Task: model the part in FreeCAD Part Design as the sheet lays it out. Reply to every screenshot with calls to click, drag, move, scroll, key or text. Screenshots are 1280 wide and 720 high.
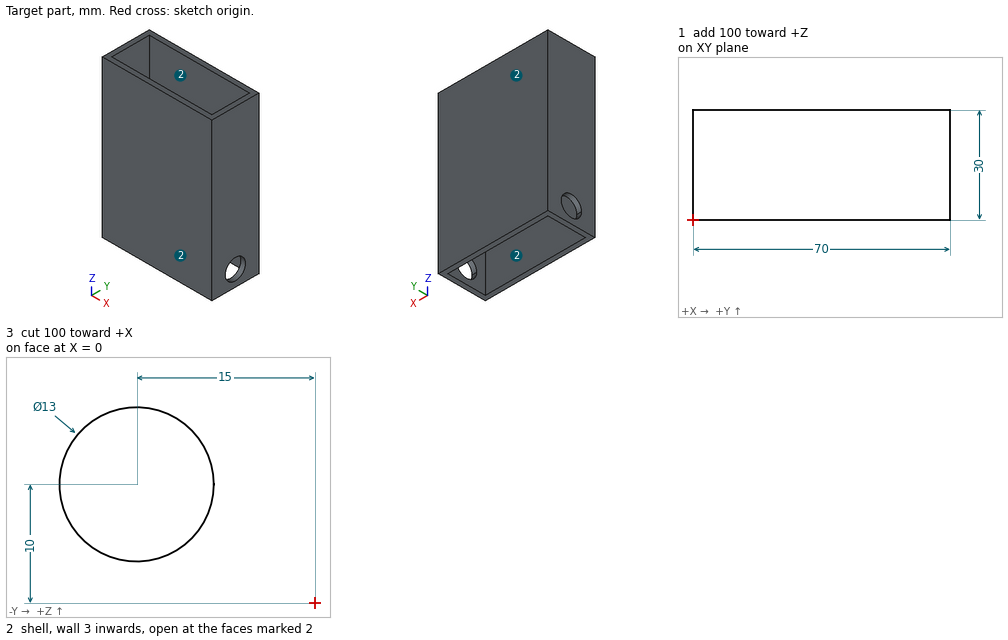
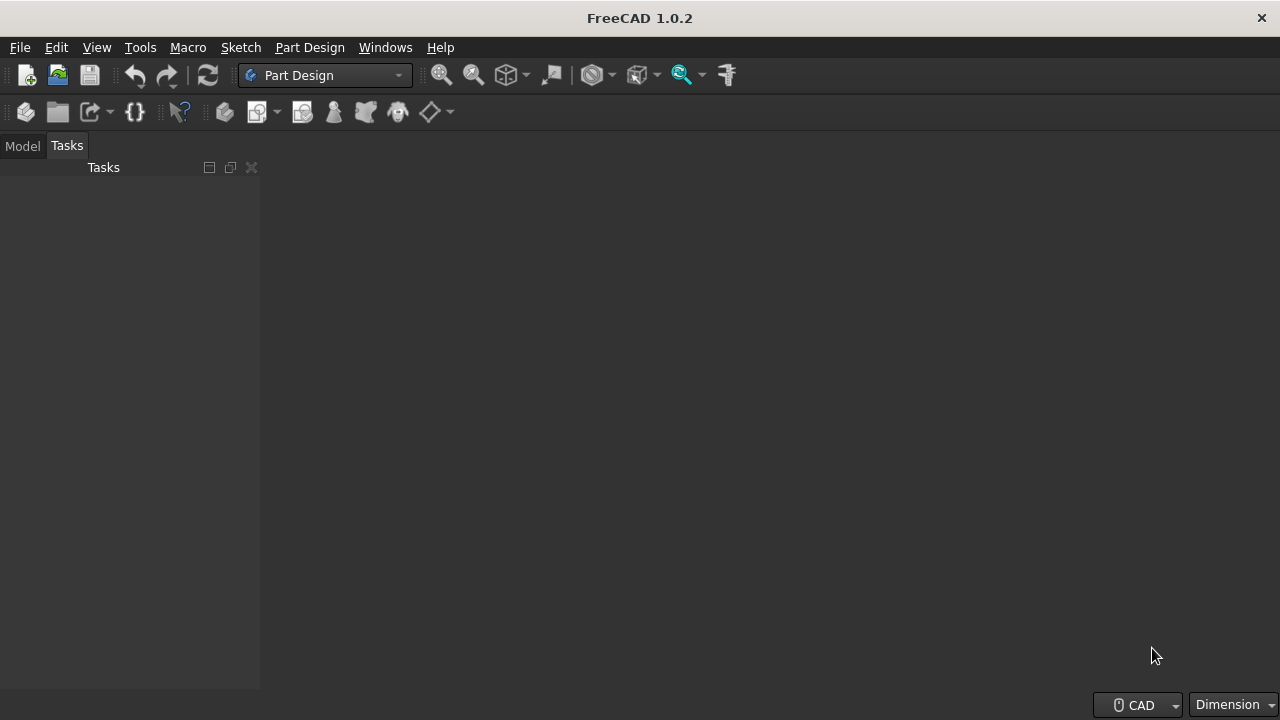
click(26, 76)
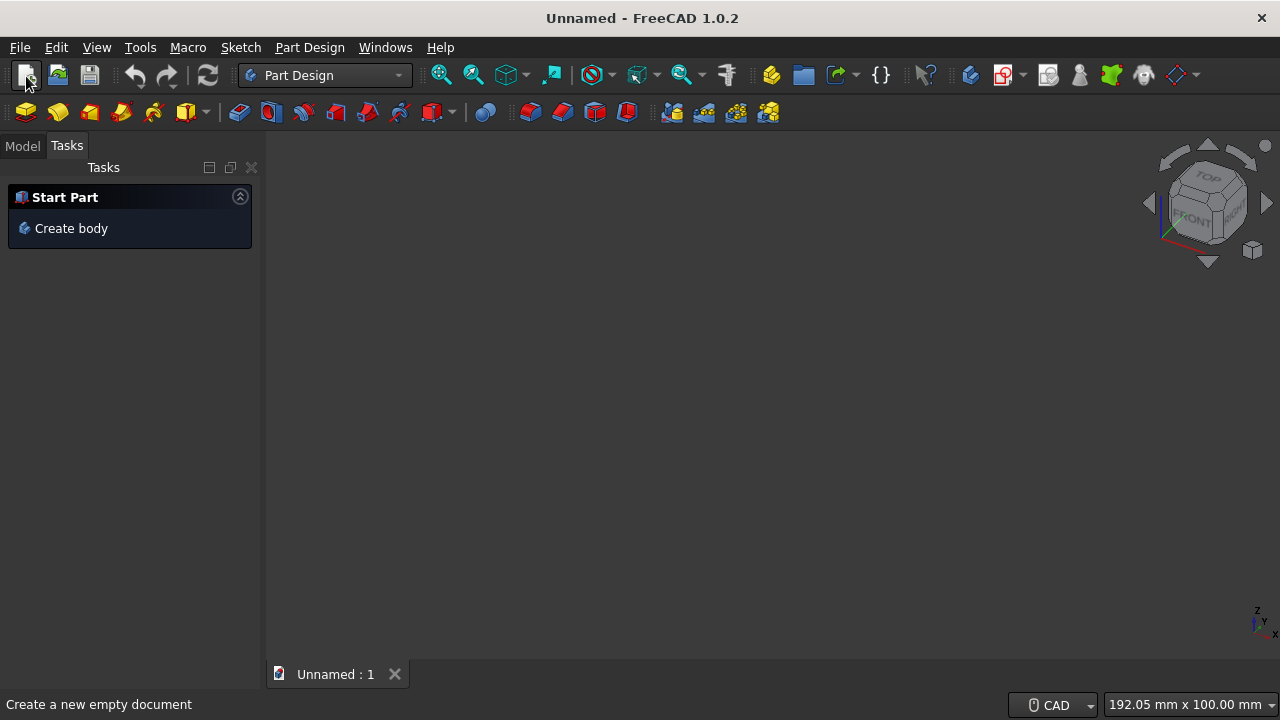
click(1004, 76)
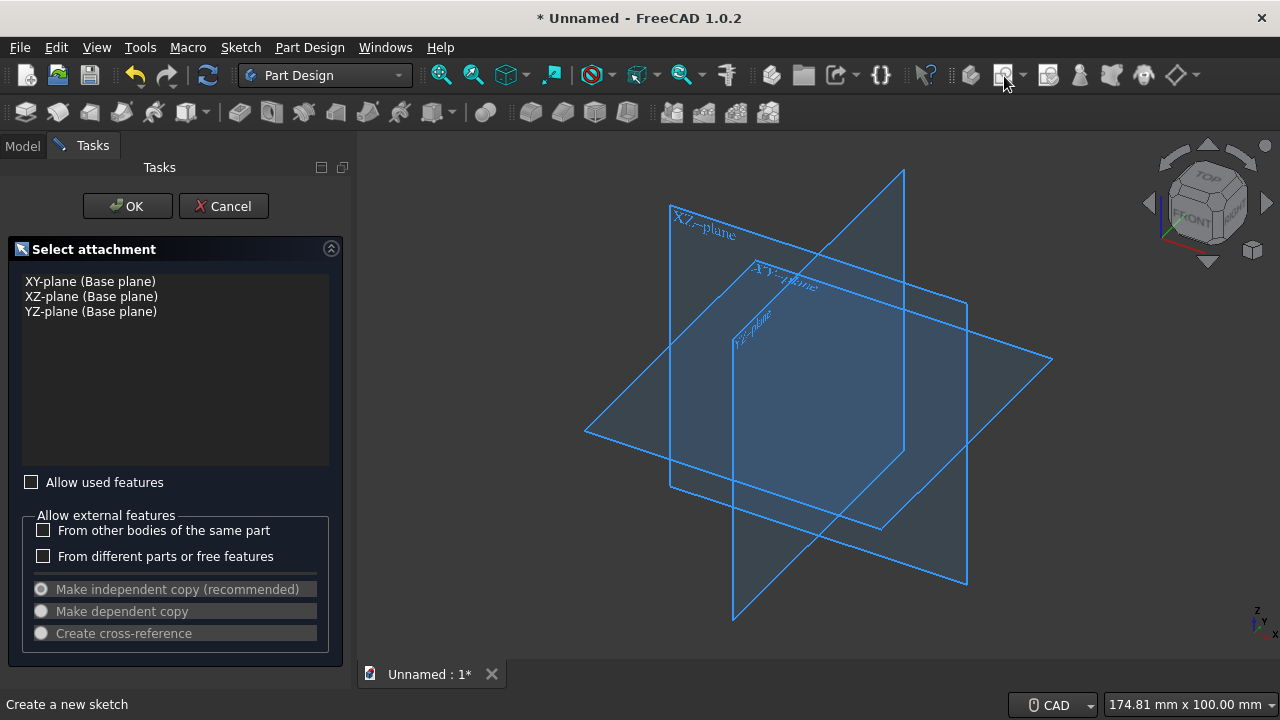
click(82, 282)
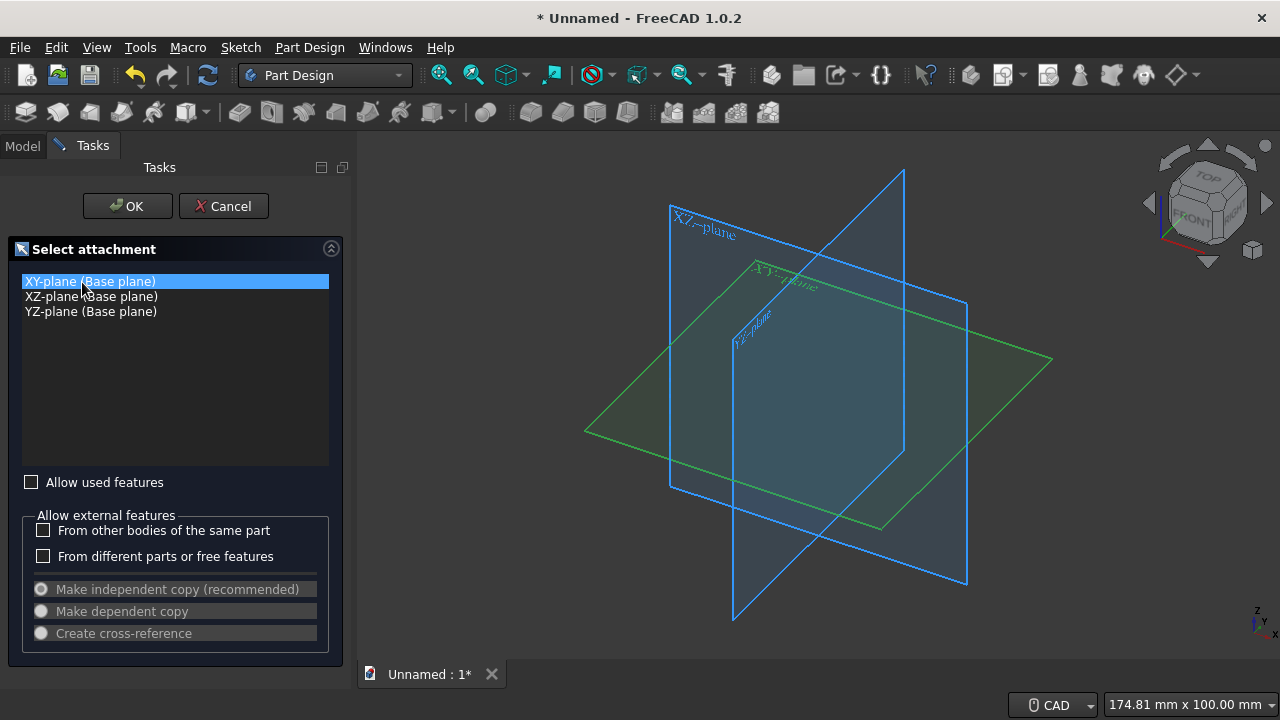
click(128, 206)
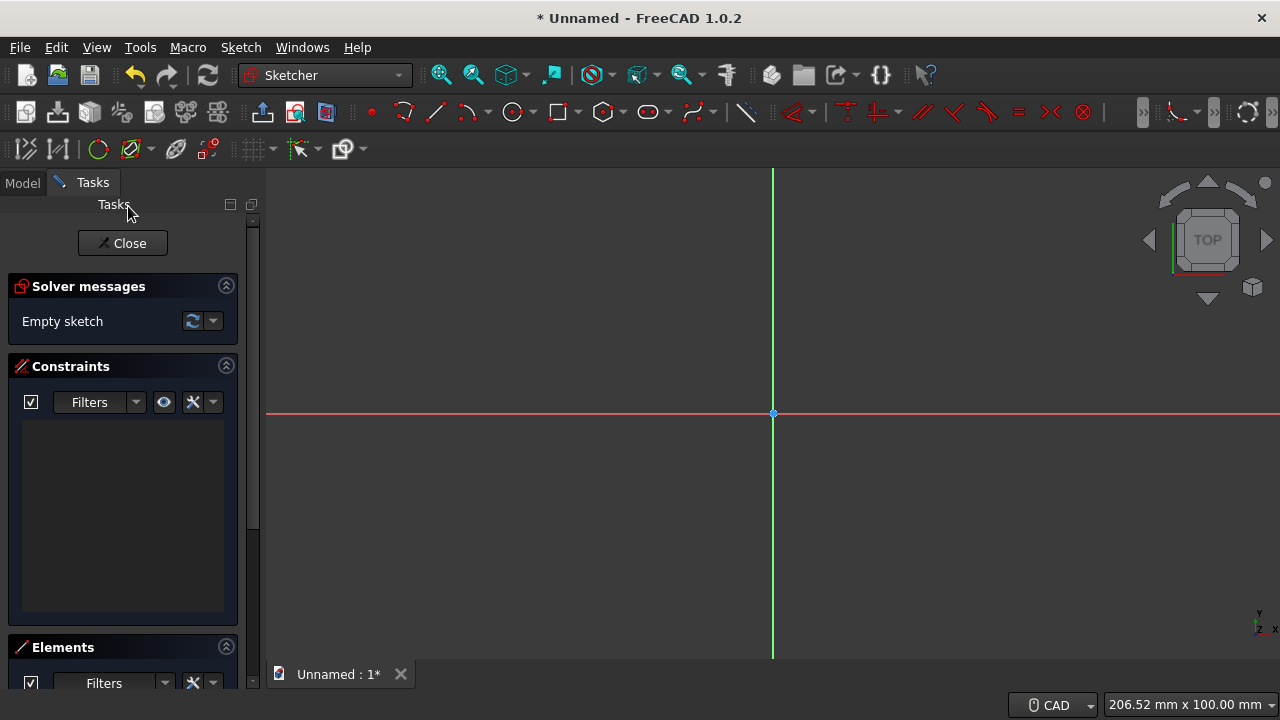
scroll(704, 414, down, 5)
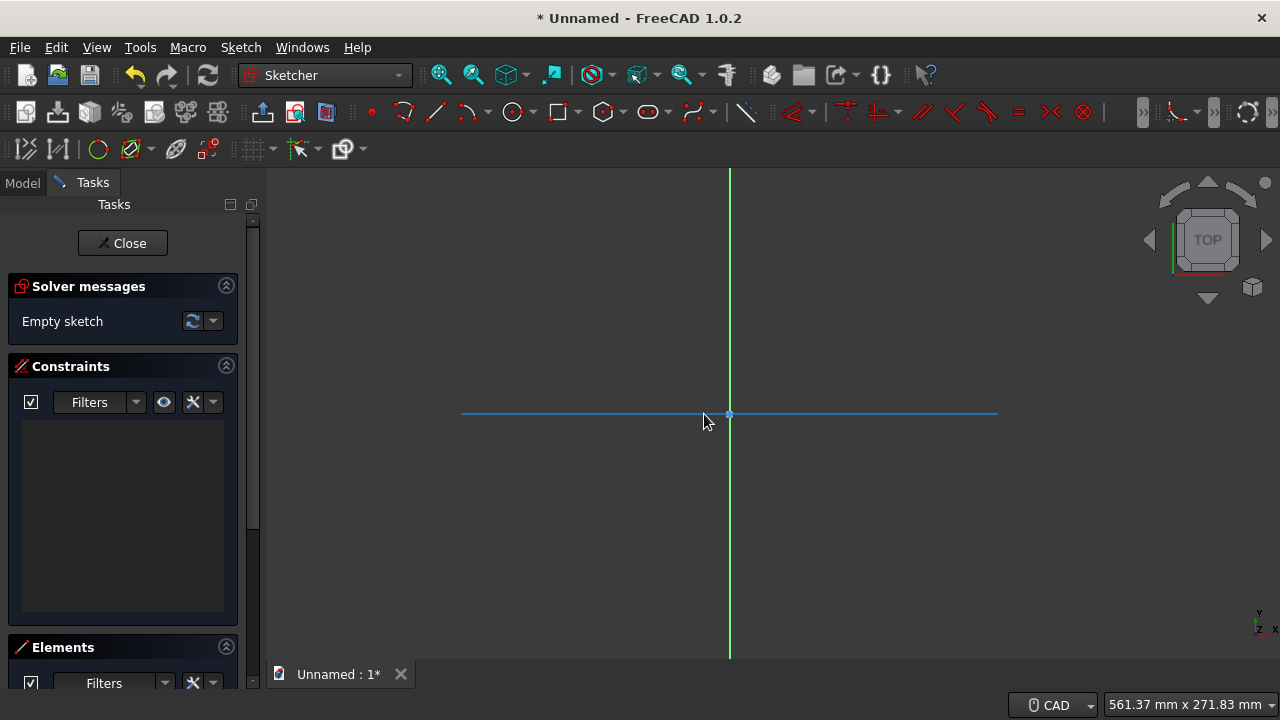
scroll(815, 380, up, 8)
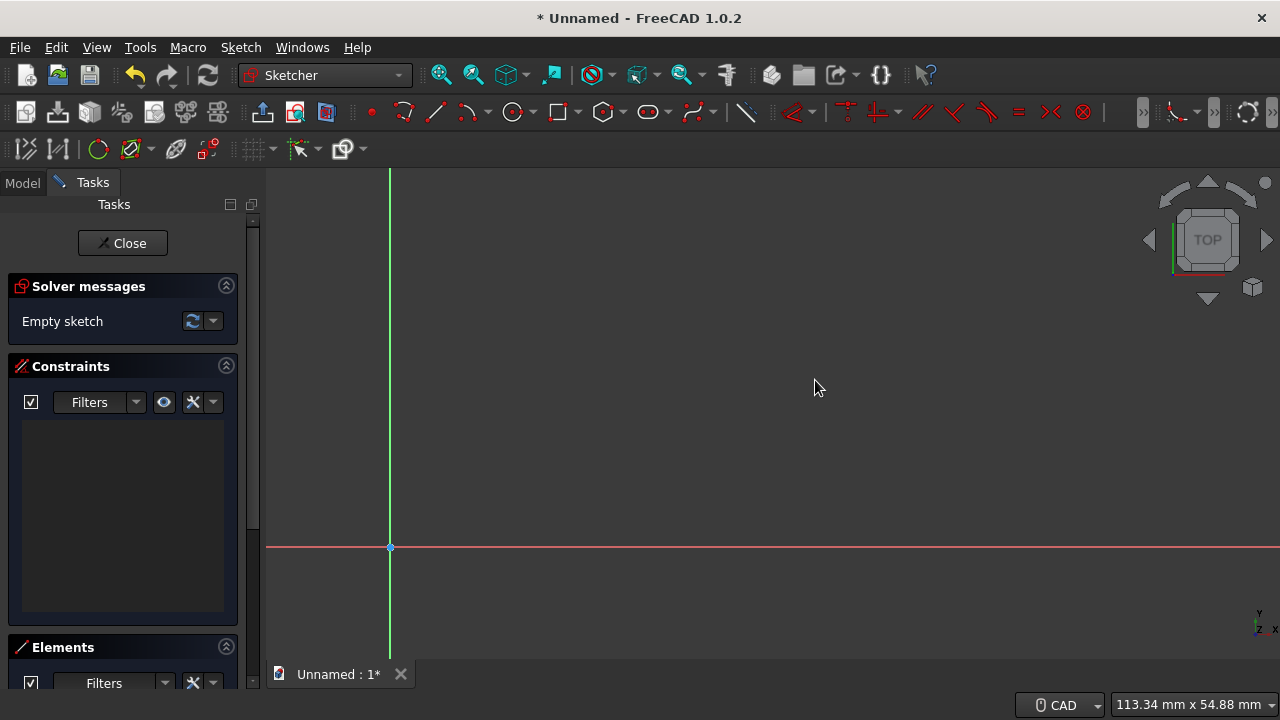
click(558, 112)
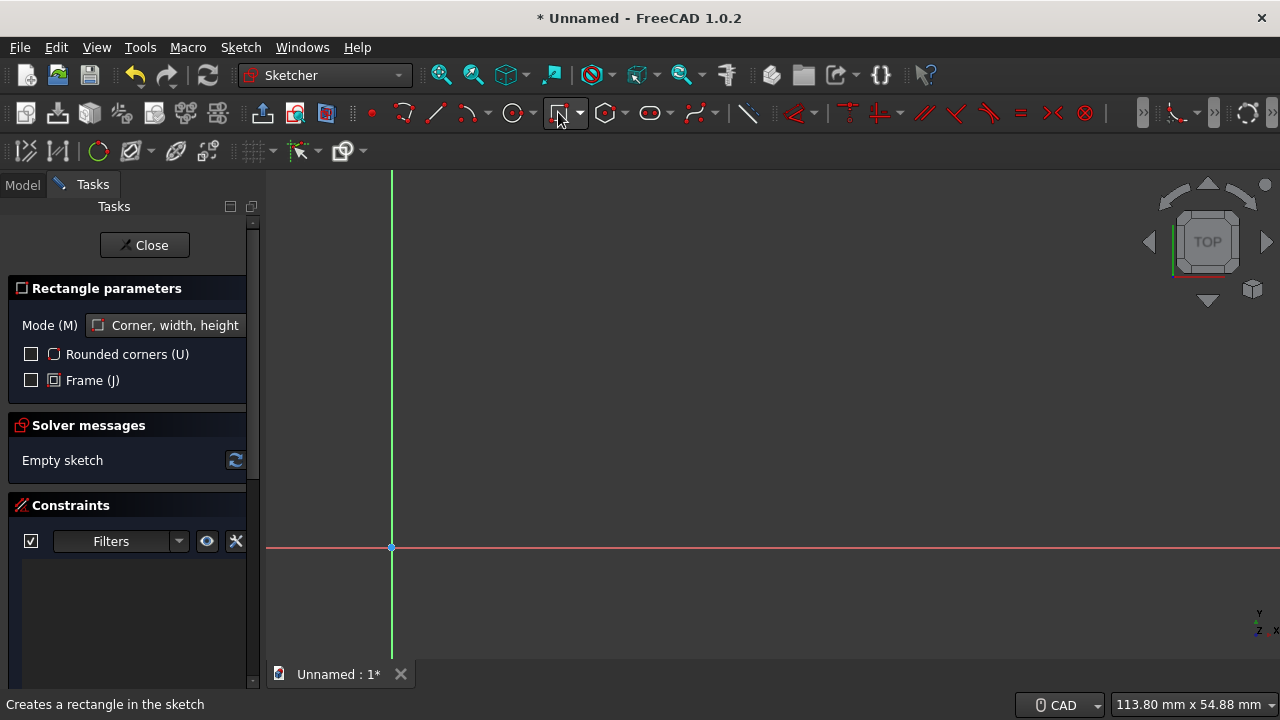
click(392, 548)
move(1015, 281)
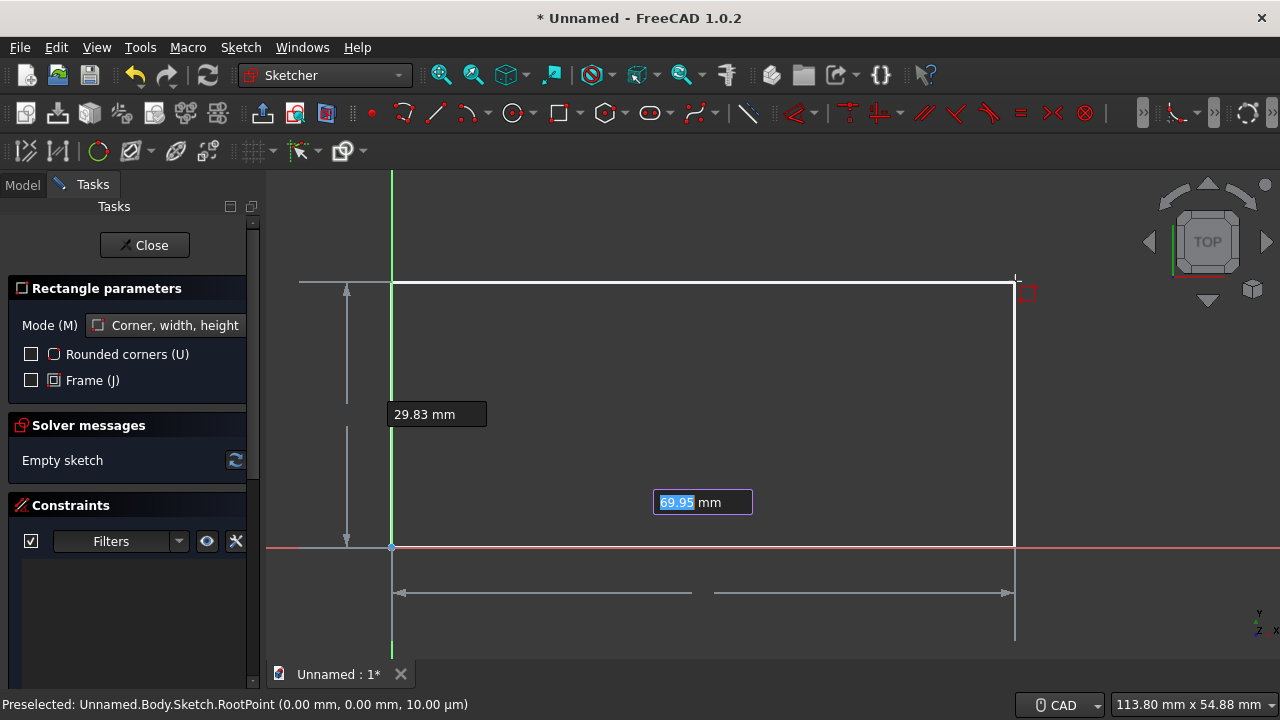
text(70)
key(Tab)
text(30)
key(Return)
key(Escape)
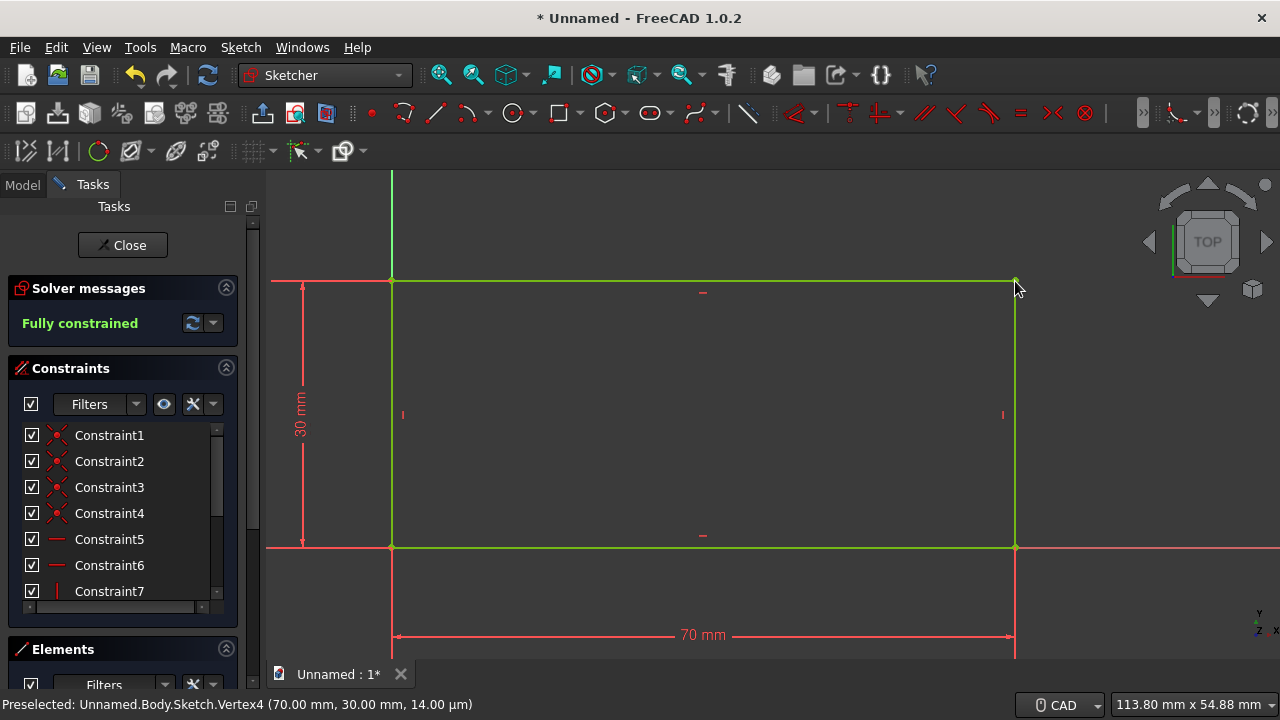
click(123, 245)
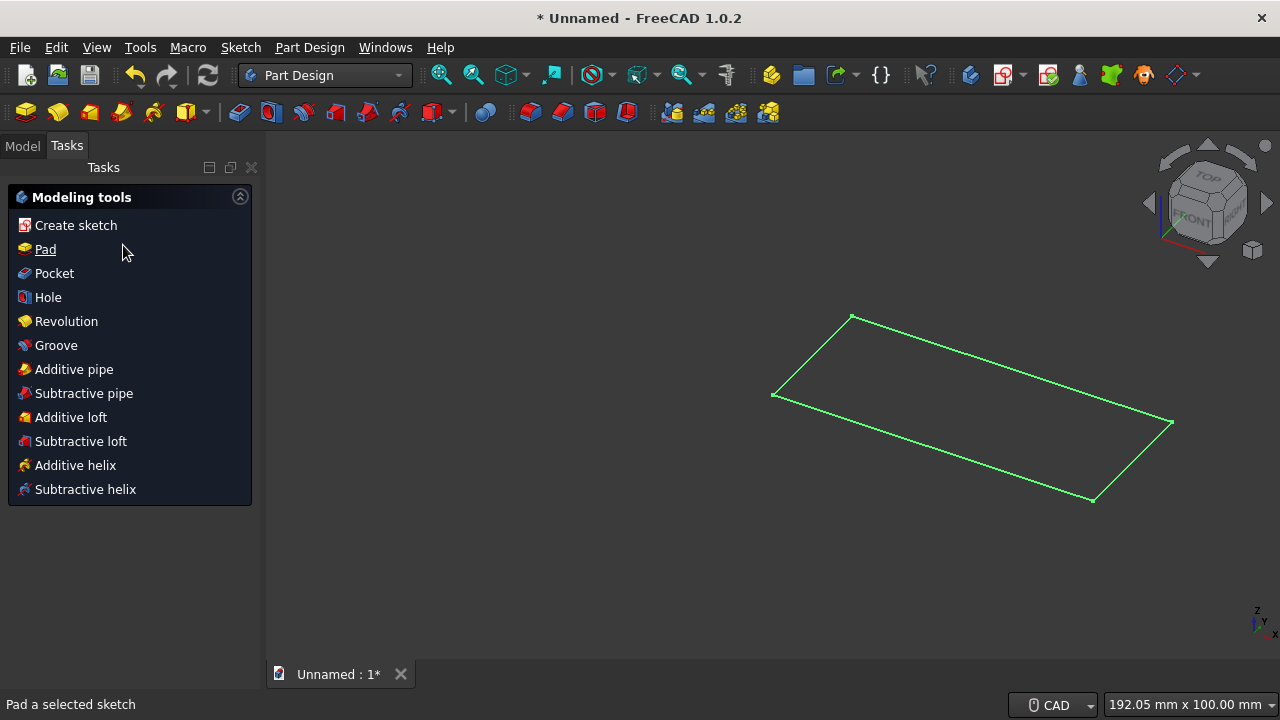
click(26, 112)